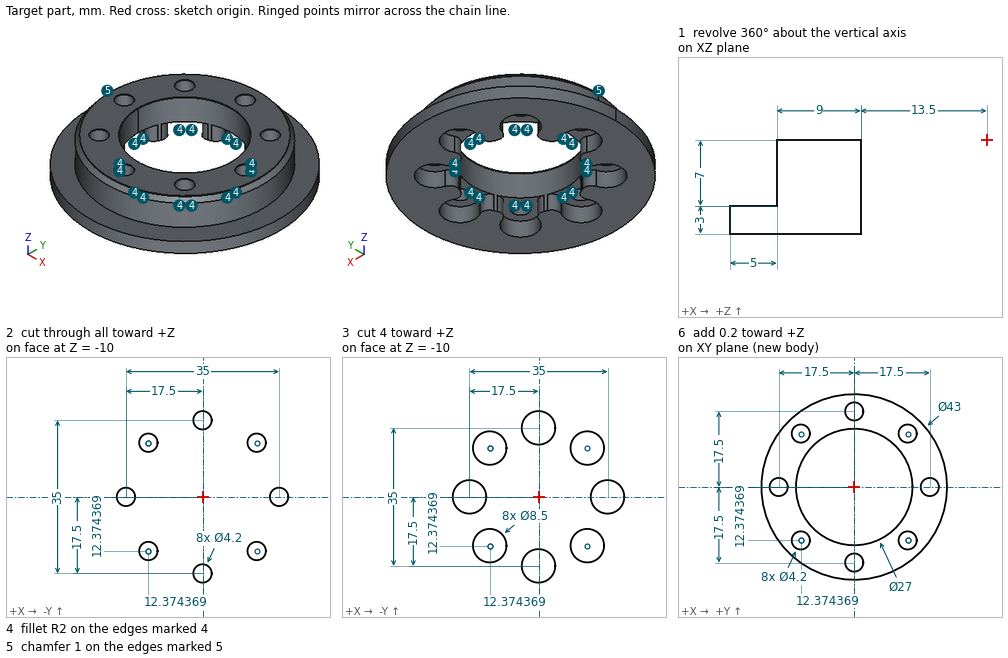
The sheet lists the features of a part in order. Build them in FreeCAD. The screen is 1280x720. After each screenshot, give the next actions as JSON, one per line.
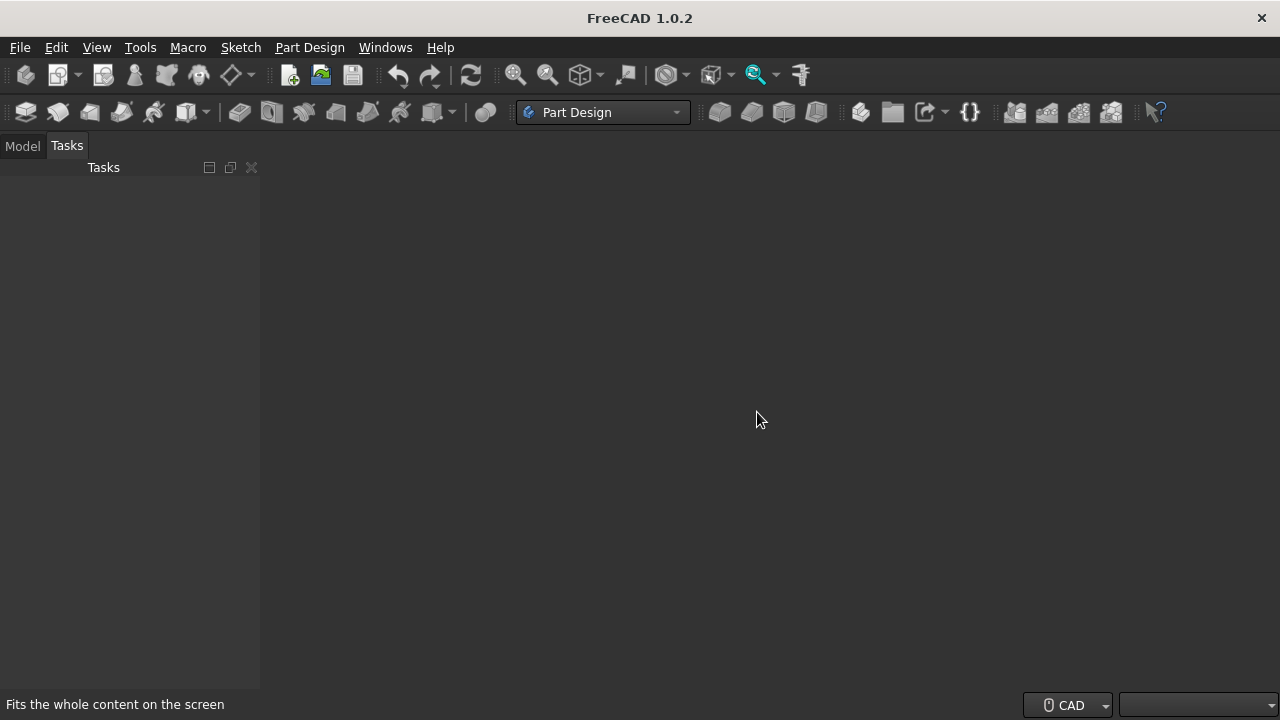
{"action": "left_click", "coordinate": [290, 76]}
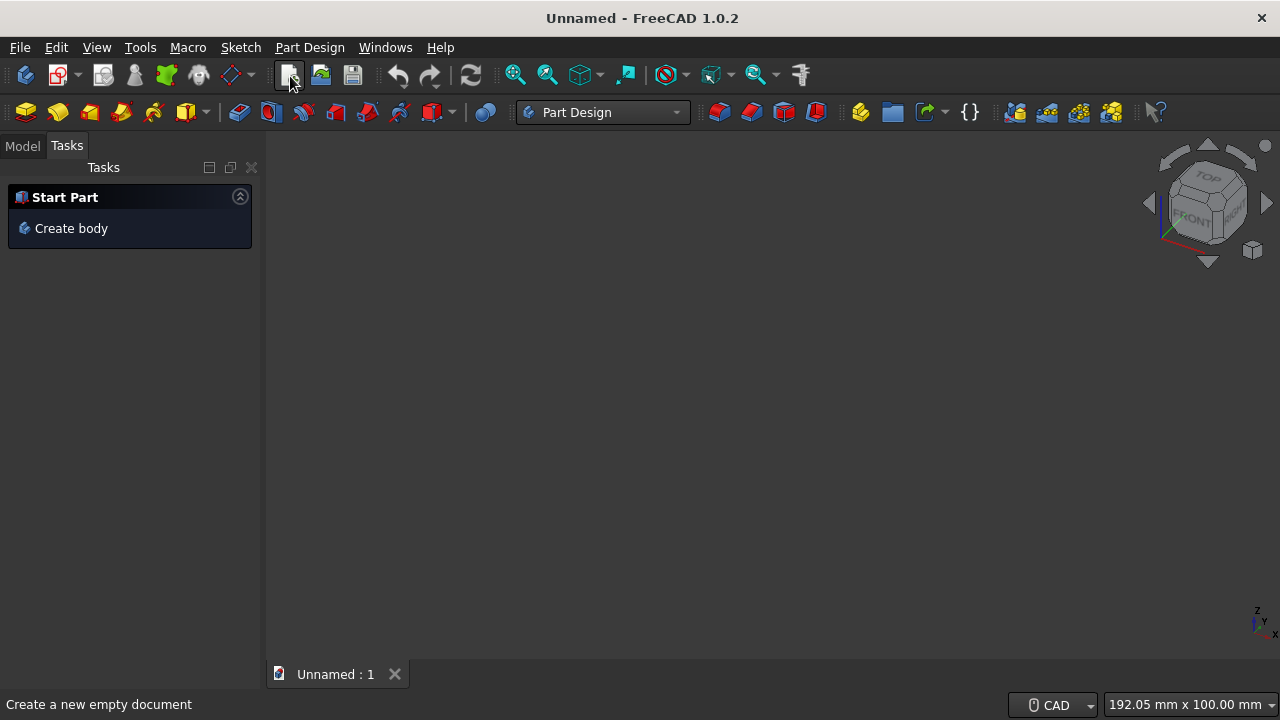
{"action": "left_click", "coordinate": [58, 76]}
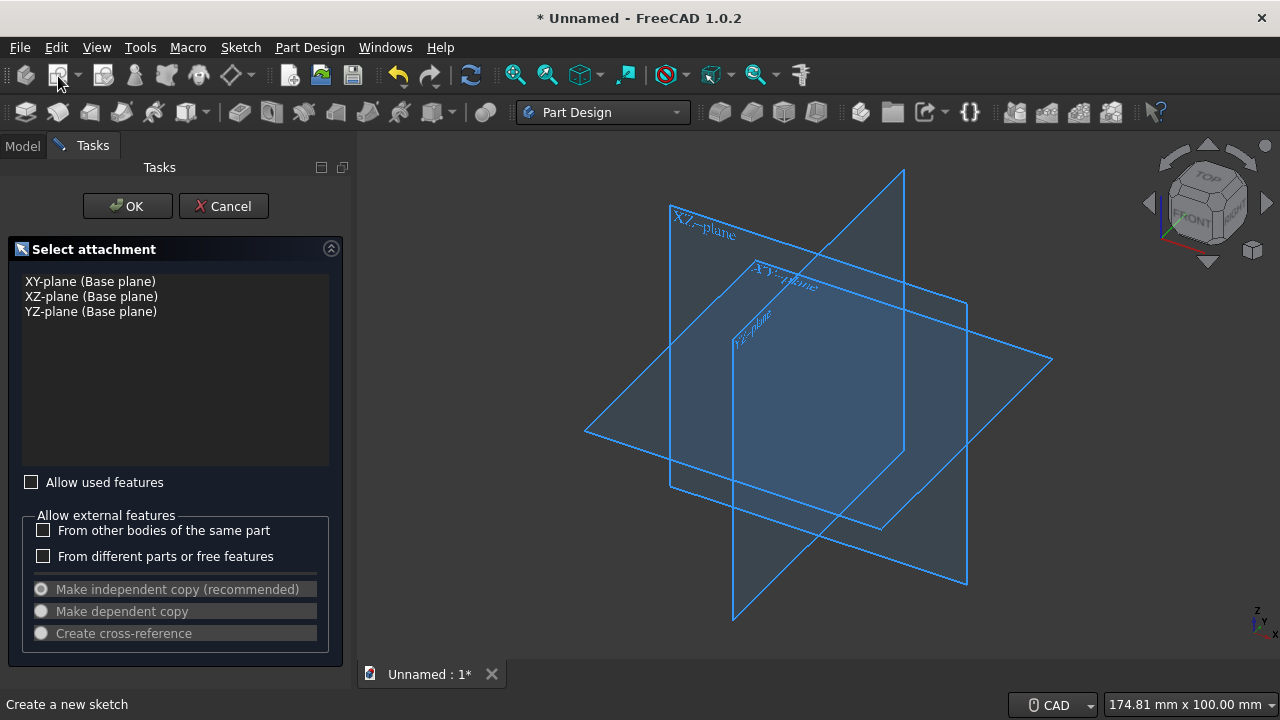
{"action": "left_click", "coordinate": [82, 296]}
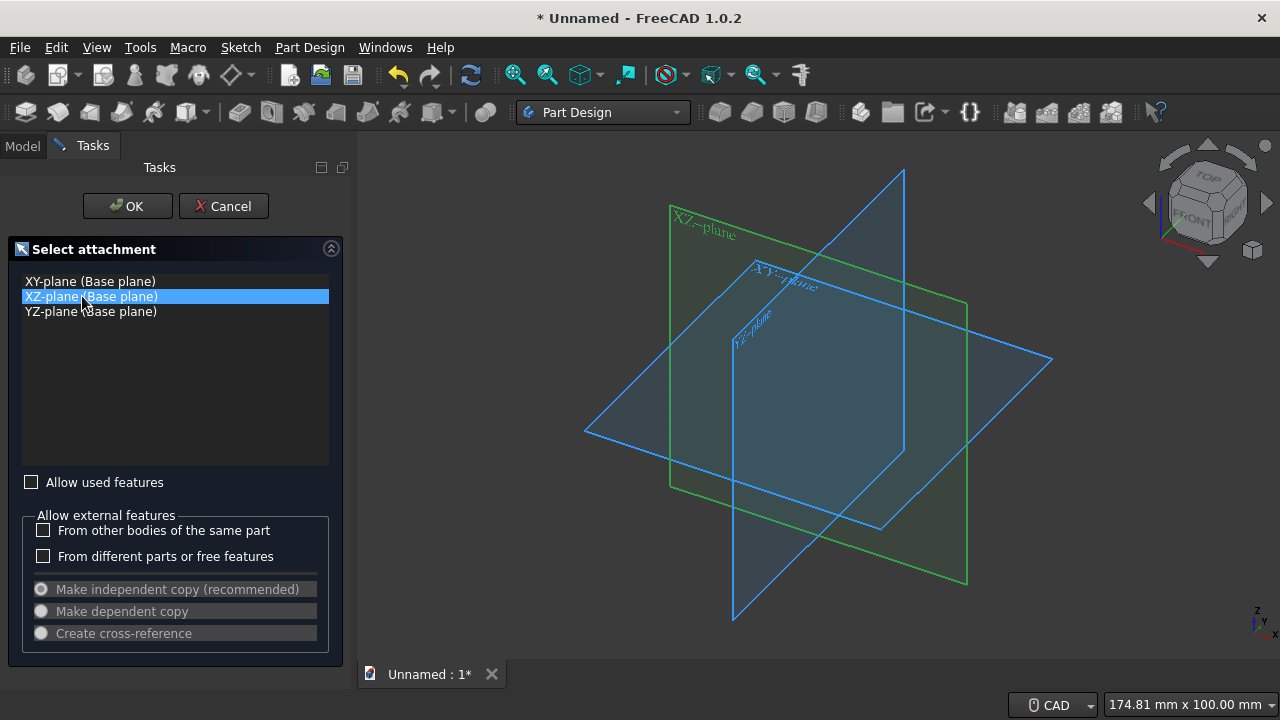
{"action": "left_click", "coordinate": [128, 206]}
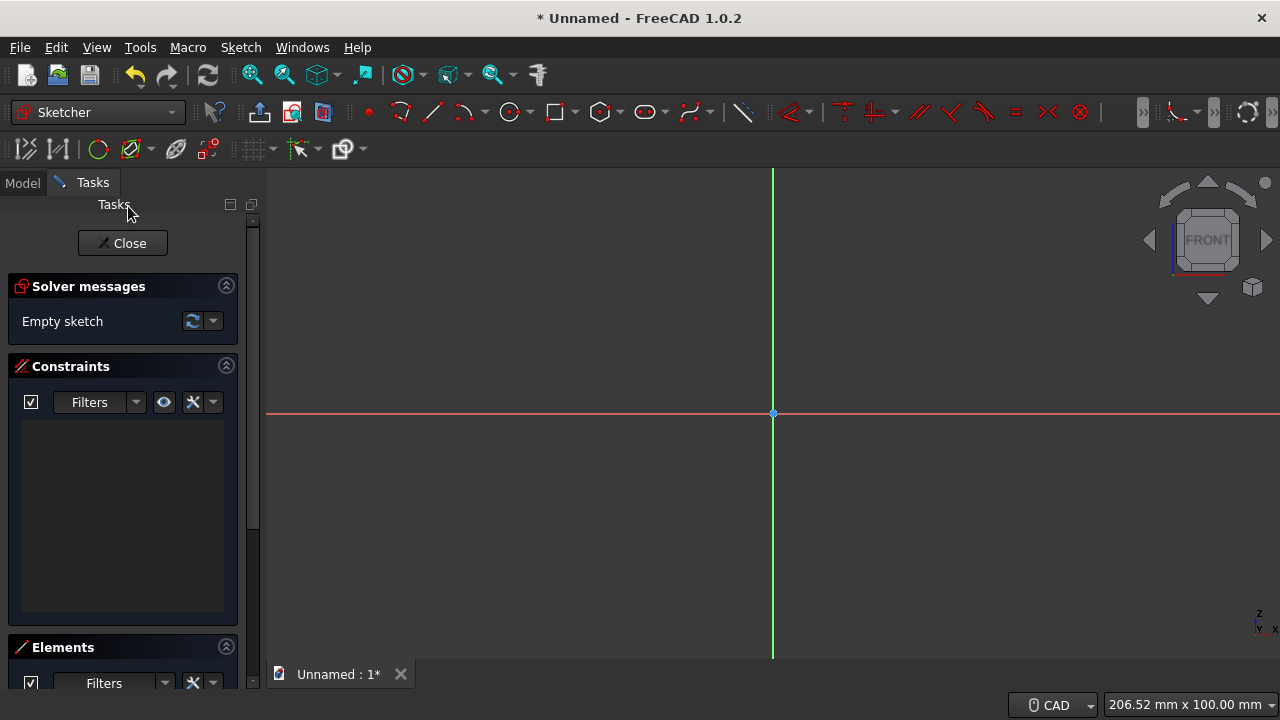
{"action": "scroll", "coordinate": [706, 446], "scroll_direction": "up", "scroll_amount": 7}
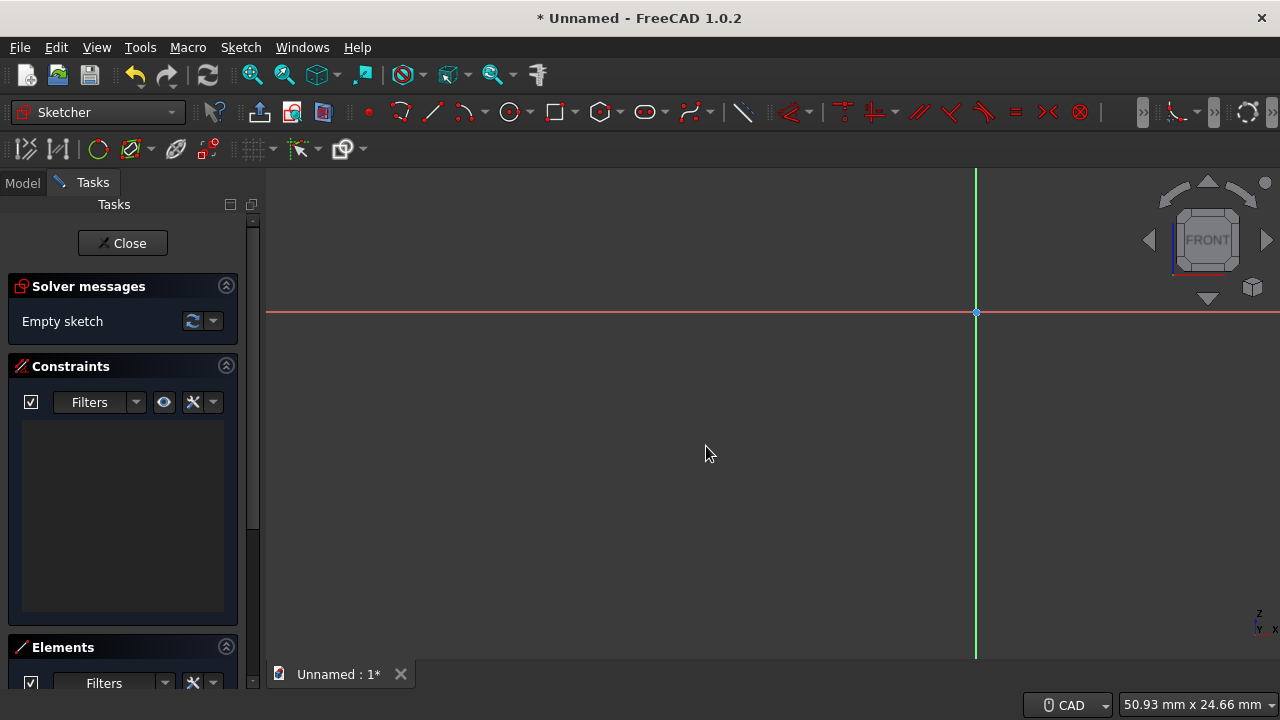
{"action": "key", "text": "g m"}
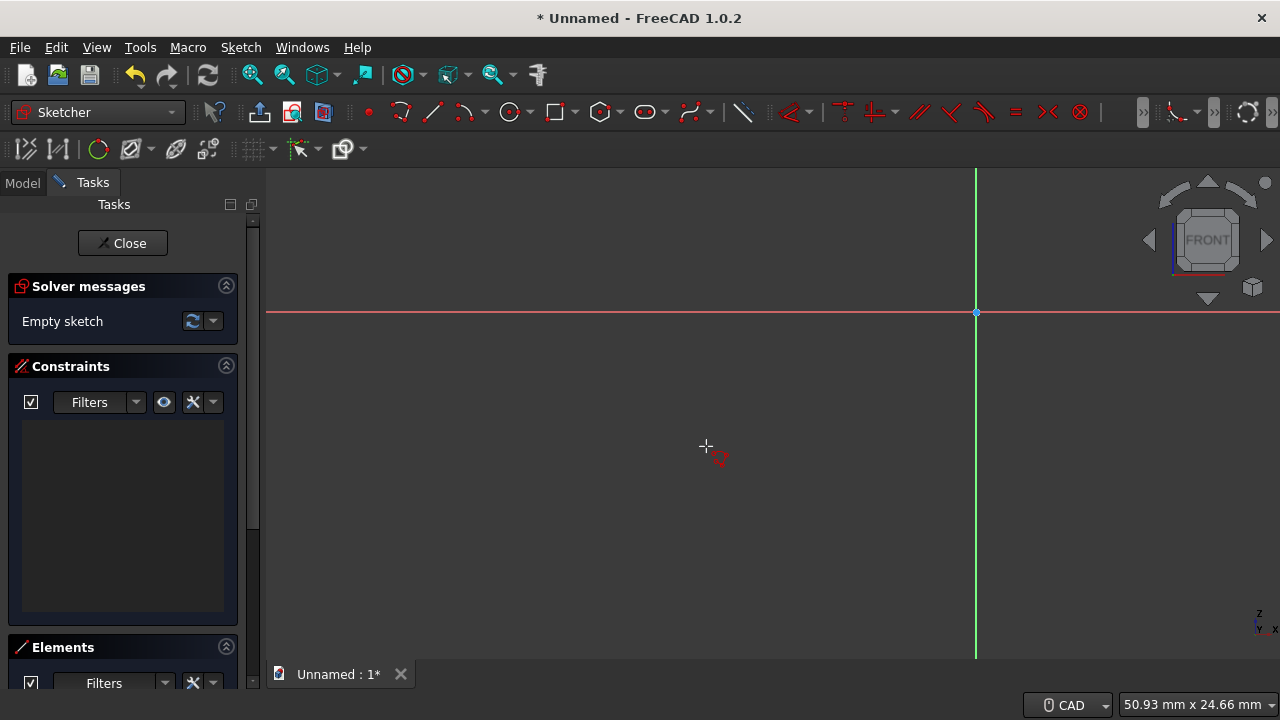
{"action": "left_click", "coordinate": [708, 312]}
{"action": "left_click", "coordinate": [708, 512]}
{"action": "left_click", "coordinate": [429, 512]}
{"action": "left_click", "coordinate": [429, 452]}
{"action": "left_click", "coordinate": [528, 452]}
{"action": "left_click", "coordinate": [528, 321]}
{"action": "left_click", "coordinate": [708, 312]}
{"action": "key", "text": "Escape"}
{"action": "key", "text": "Escape"}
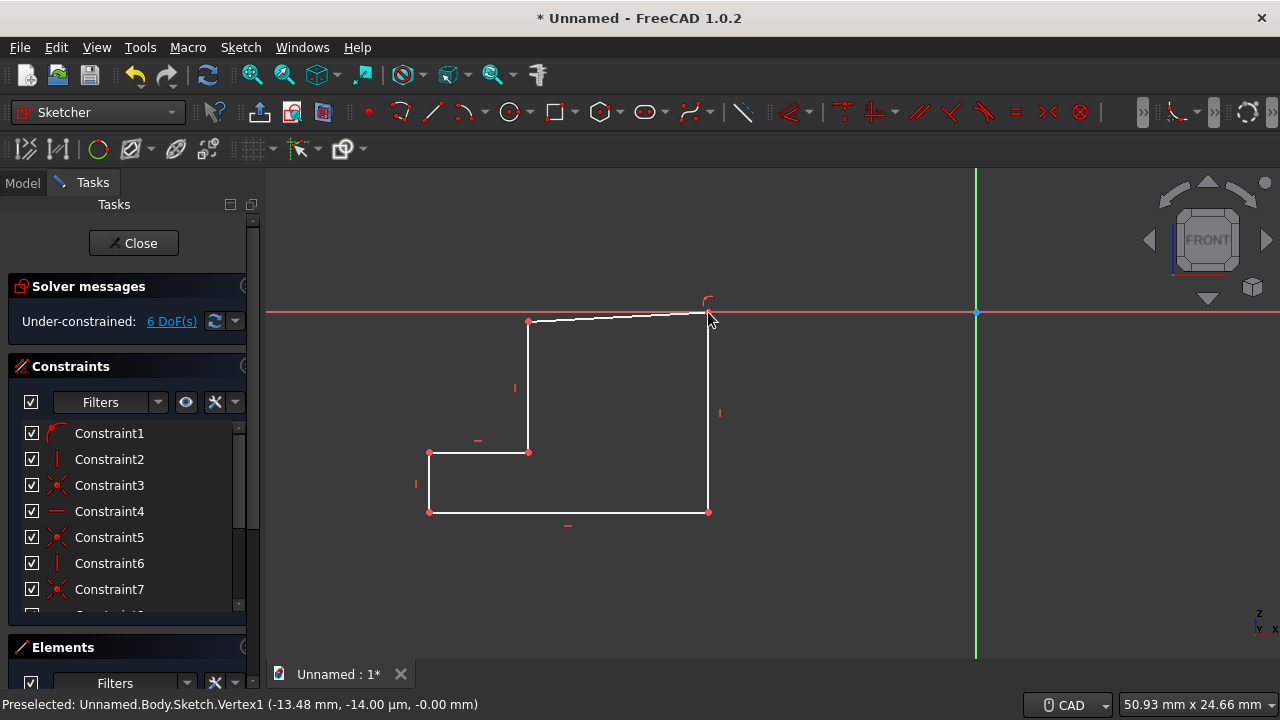
{"action": "left_click", "coordinate": [654, 315]}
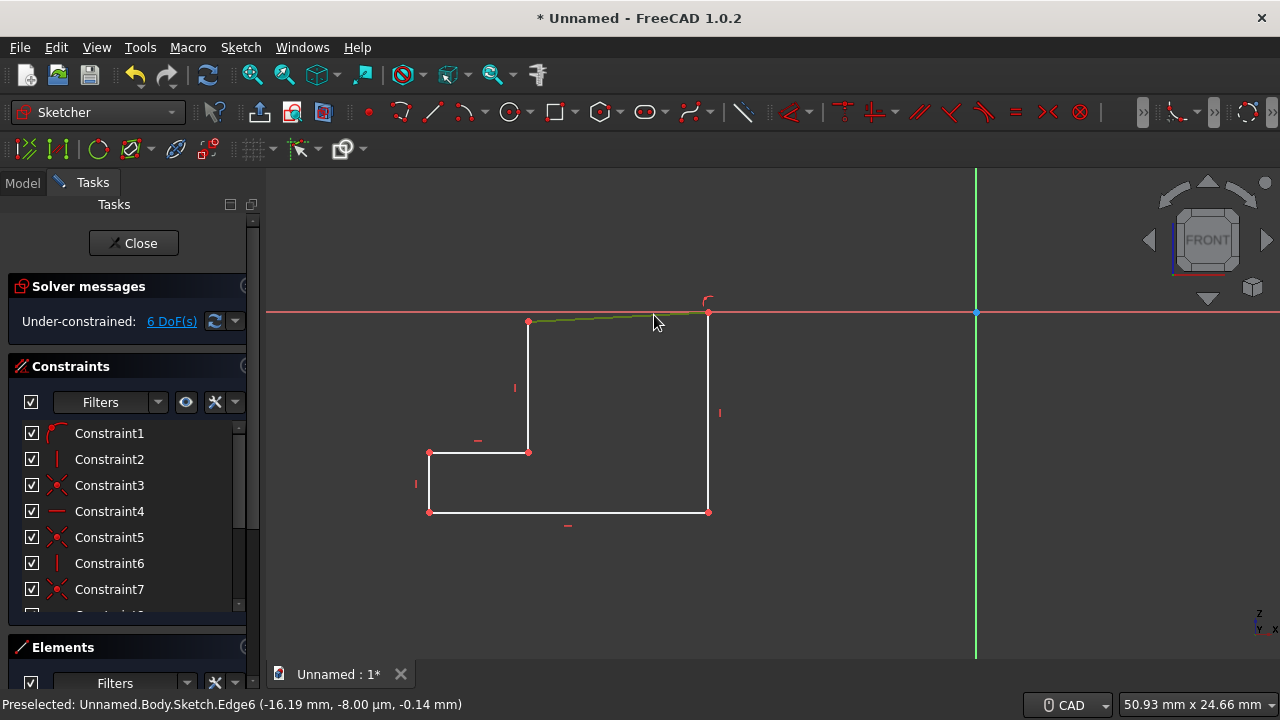
{"action": "key", "text": "h"}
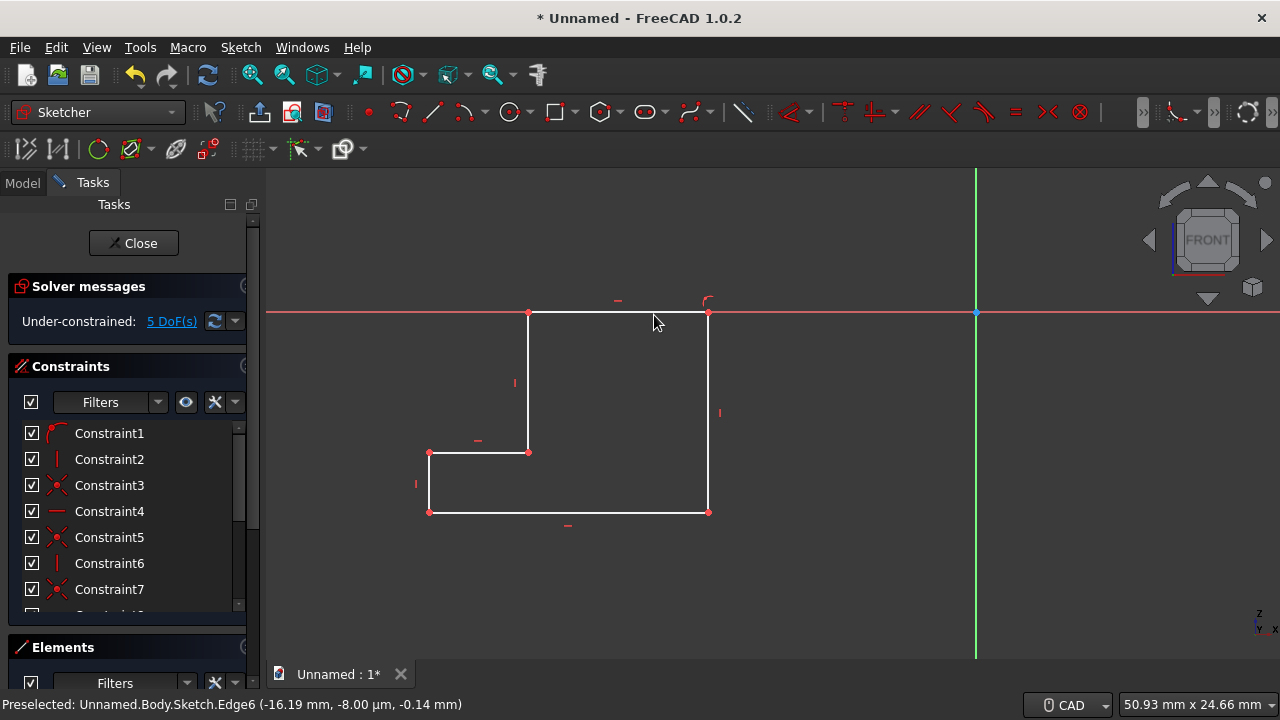
{"action": "left_click", "coordinate": [429, 495]}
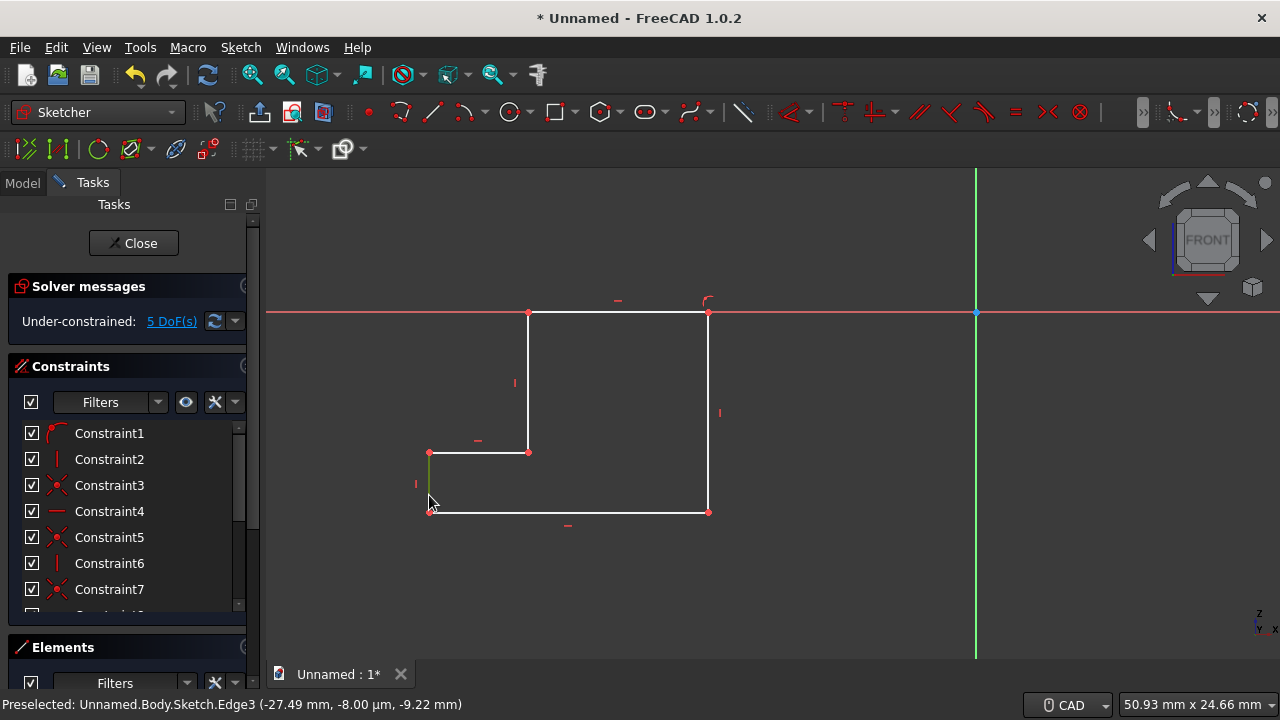
{"action": "key", "text": "i"}